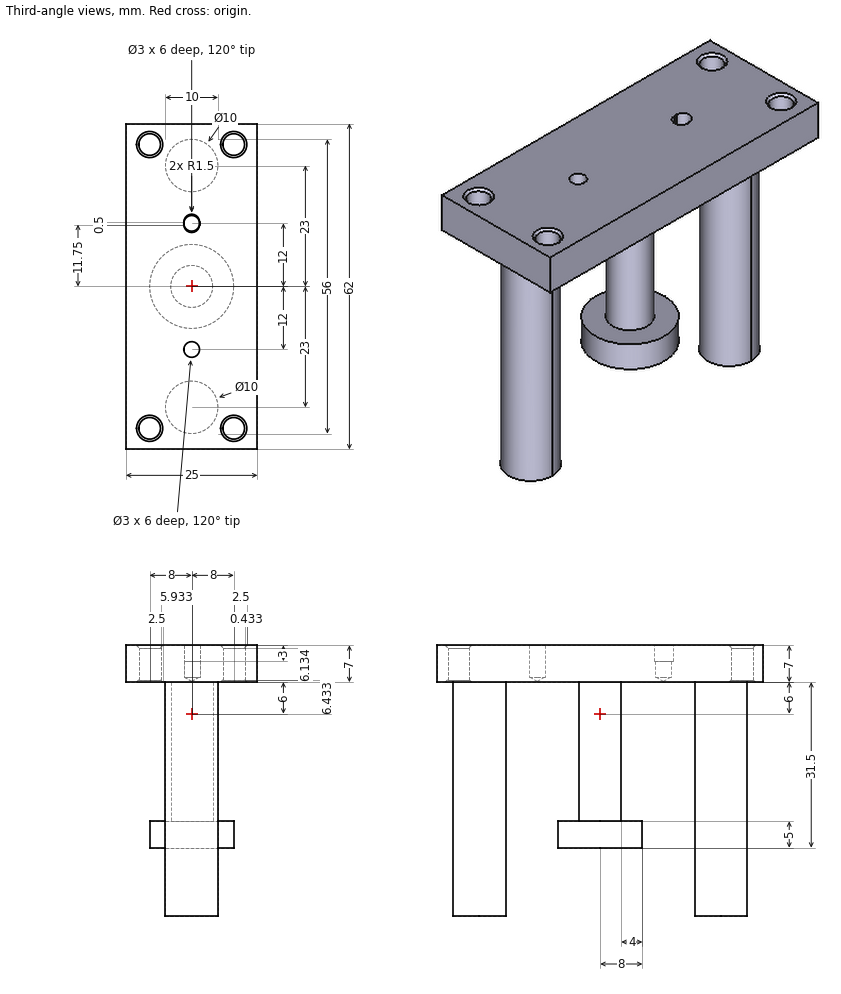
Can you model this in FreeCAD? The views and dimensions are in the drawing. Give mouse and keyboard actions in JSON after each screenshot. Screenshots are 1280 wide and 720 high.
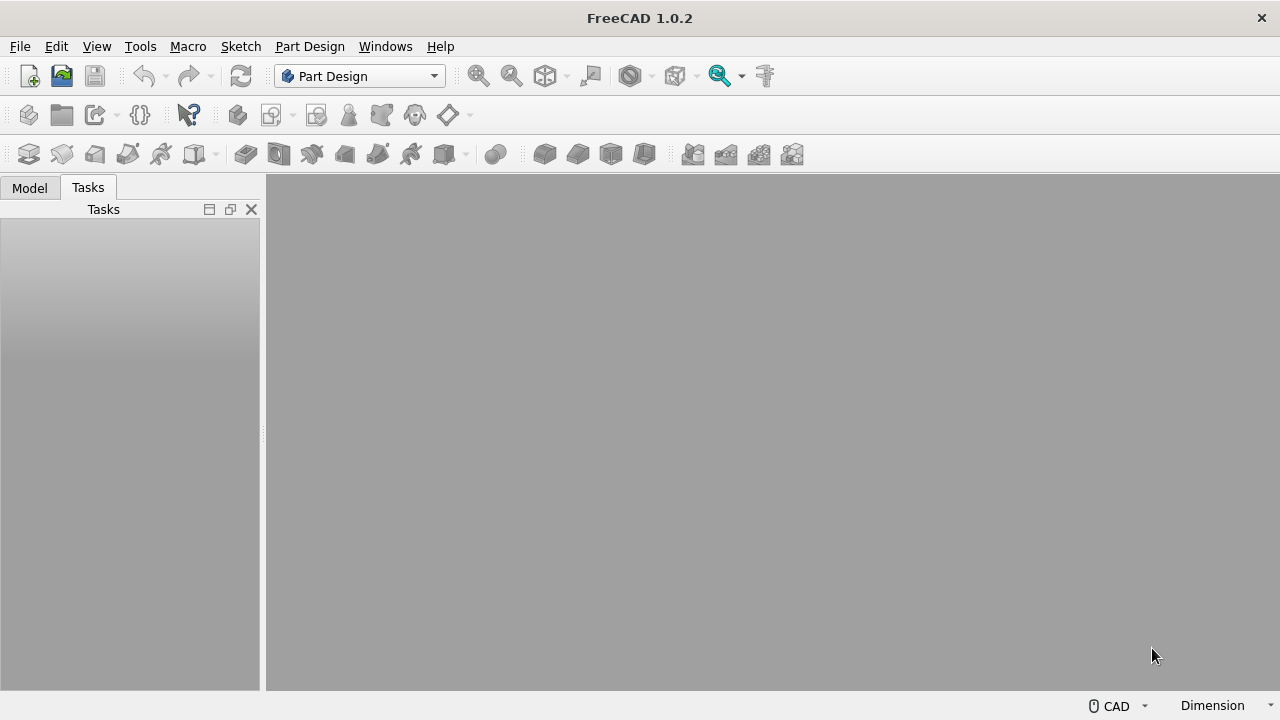
{"action": "left_click", "coordinate": [29, 76]}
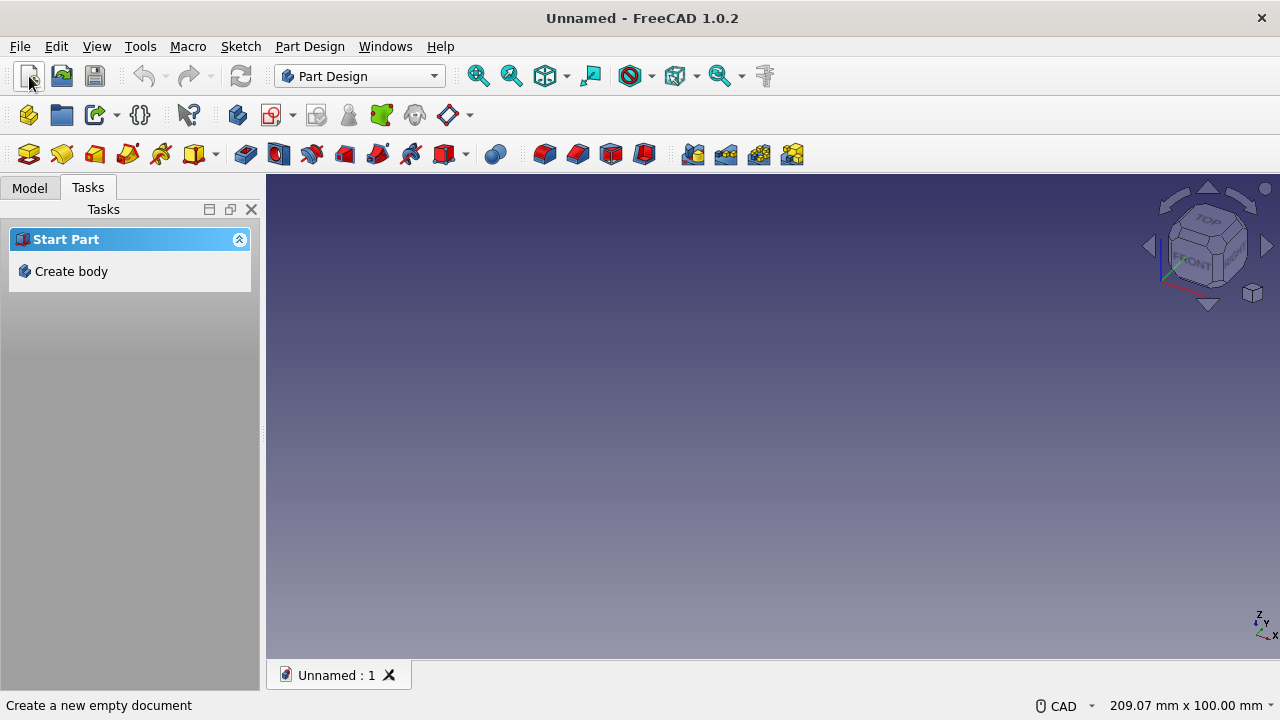
{"action": "left_click", "coordinate": [238, 116]}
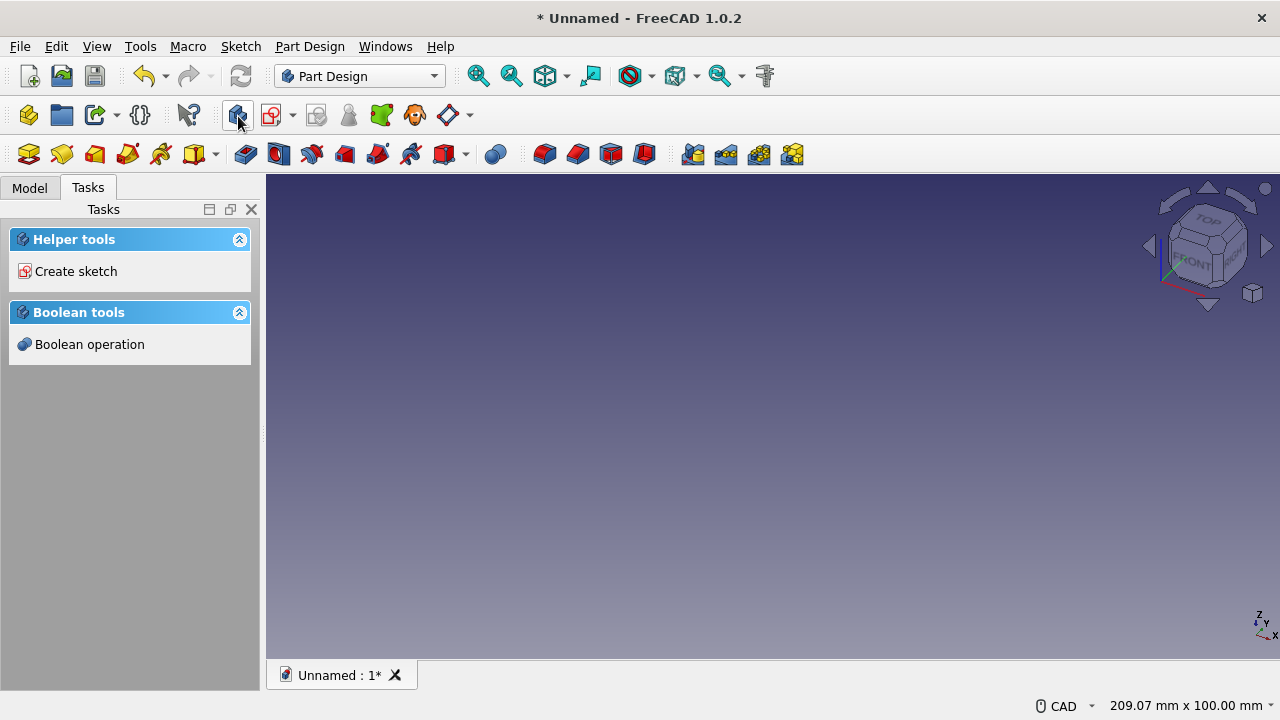
{"action": "left_click", "coordinate": [30, 188]}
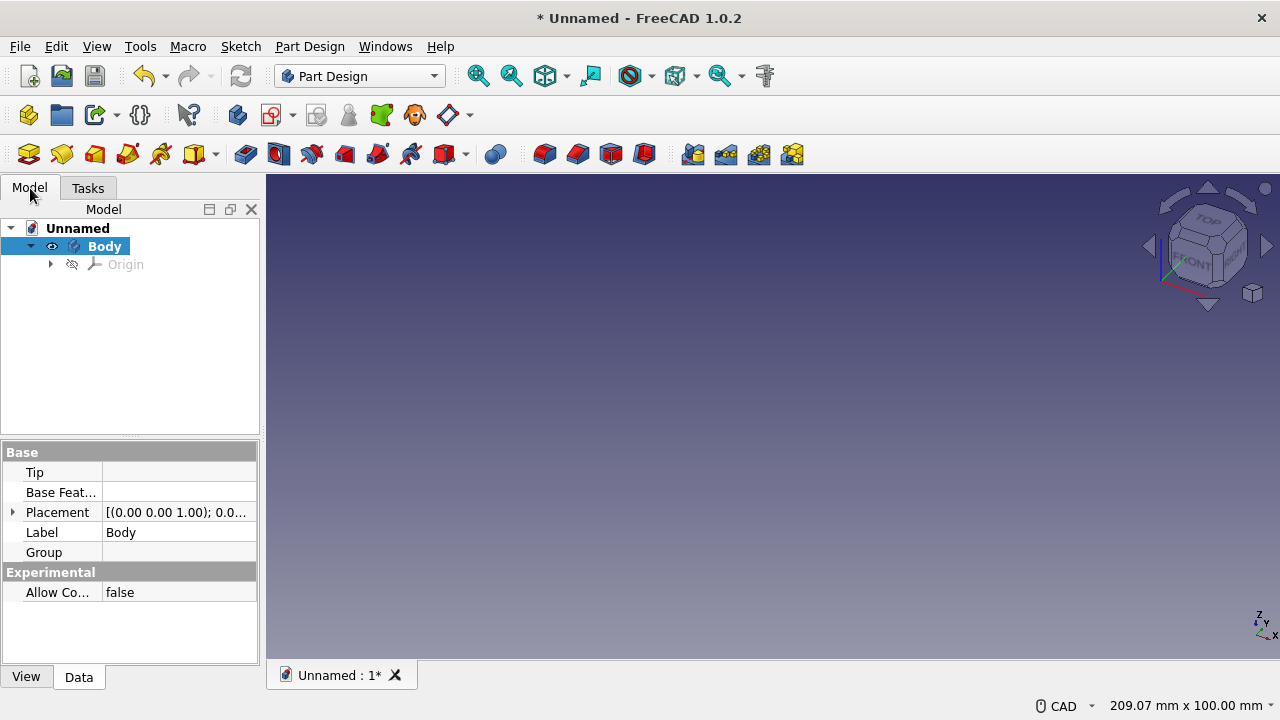
{"action": "left_click", "coordinate": [51, 264]}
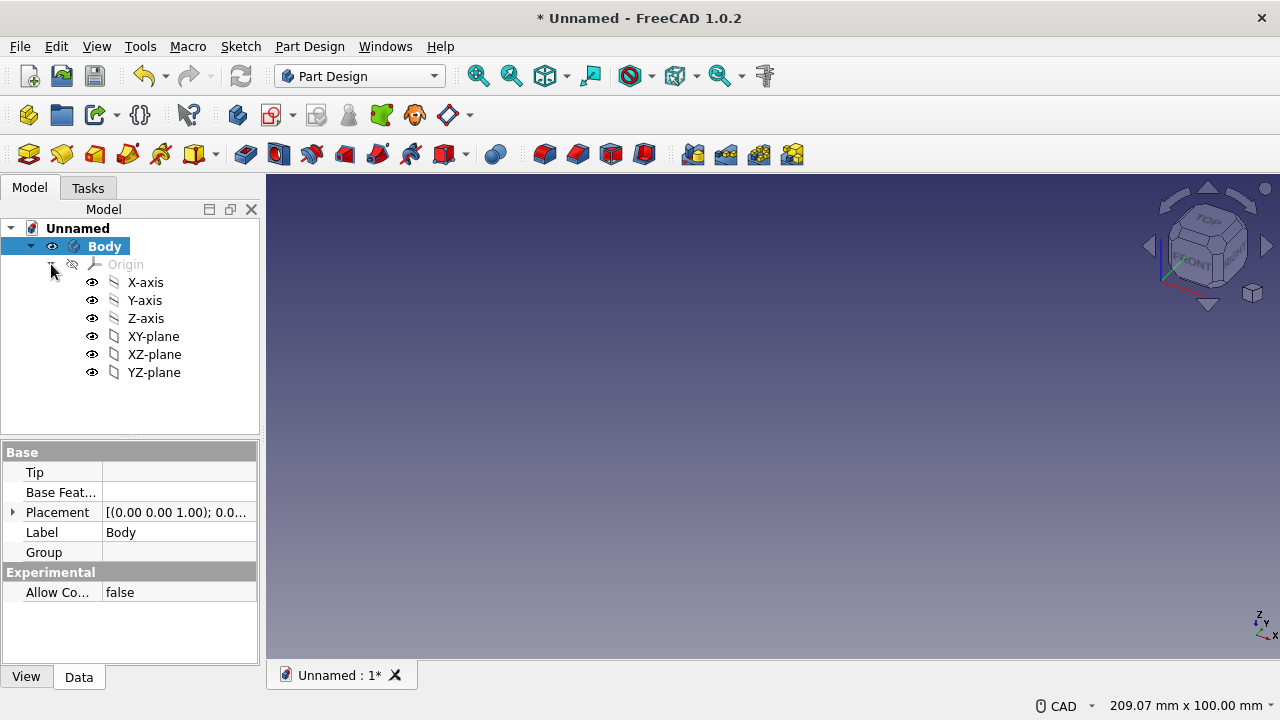
{"action": "left_click", "coordinate": [137, 336]}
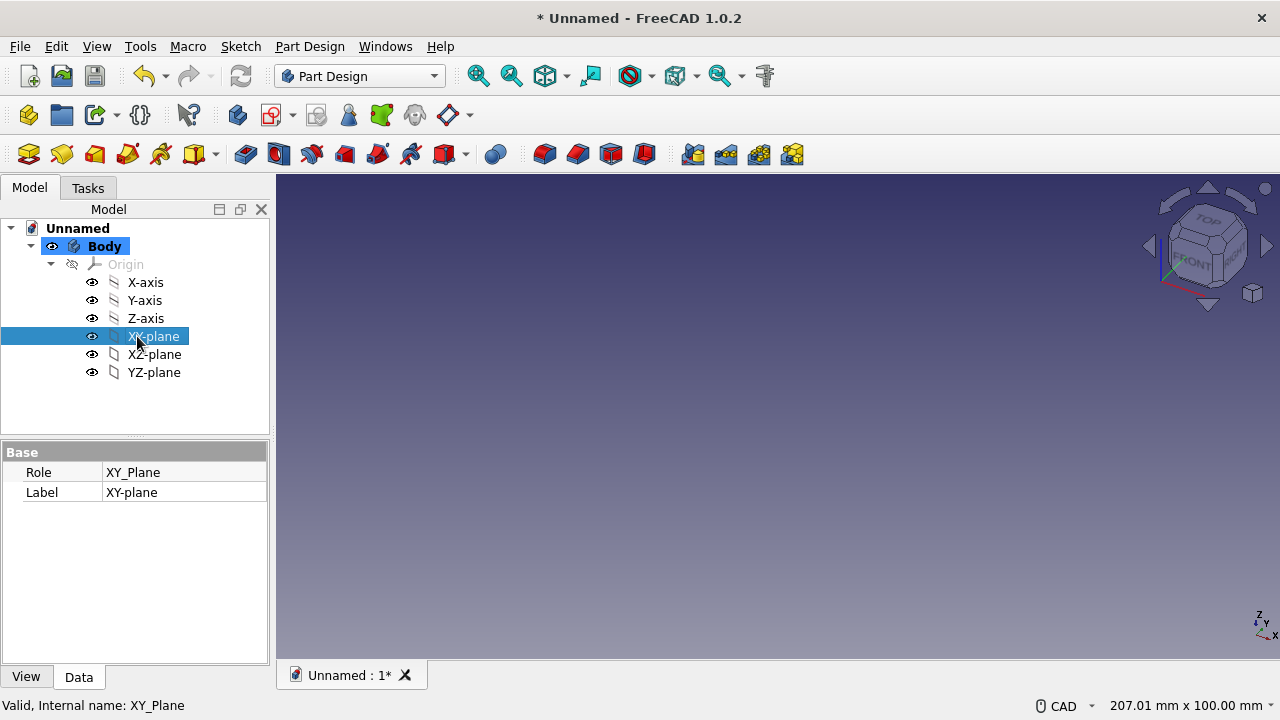
{"action": "left_click", "coordinate": [448, 116]}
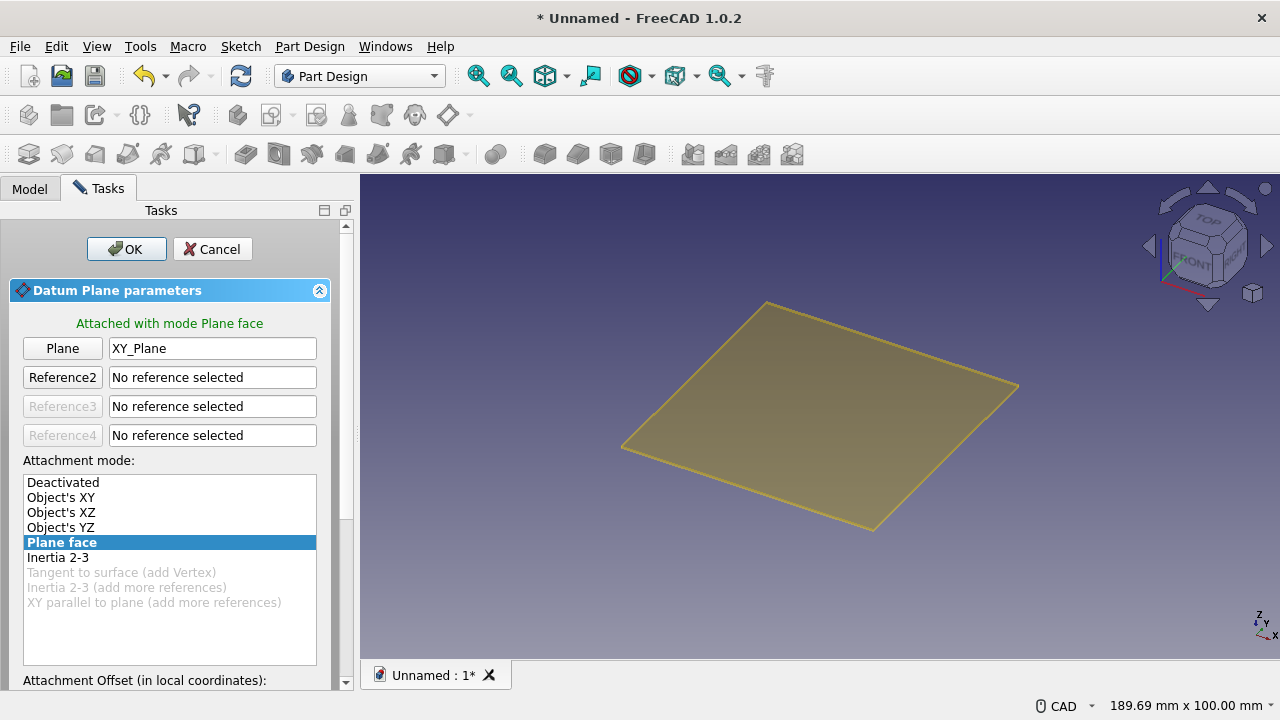
{"action": "scroll", "coordinate": [346, 455], "scroll_direction": "down", "scroll_amount": 3}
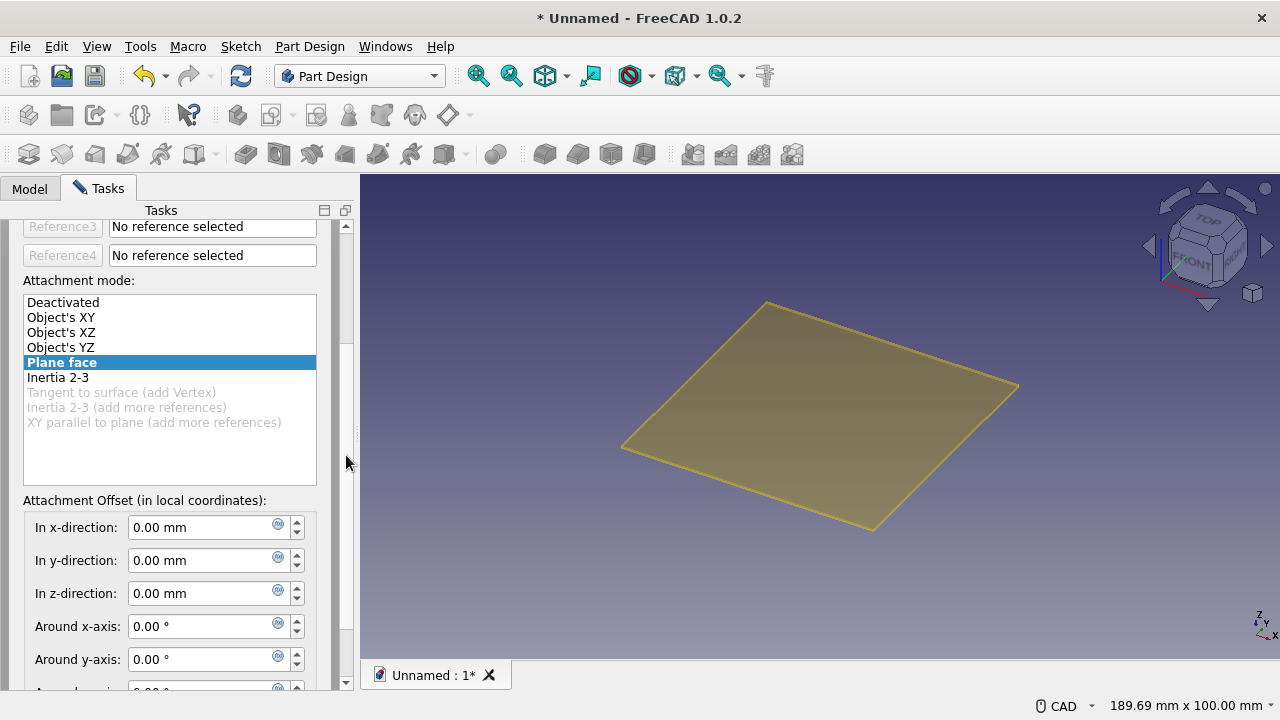
{"action": "triple_click", "coordinate": [210, 594]}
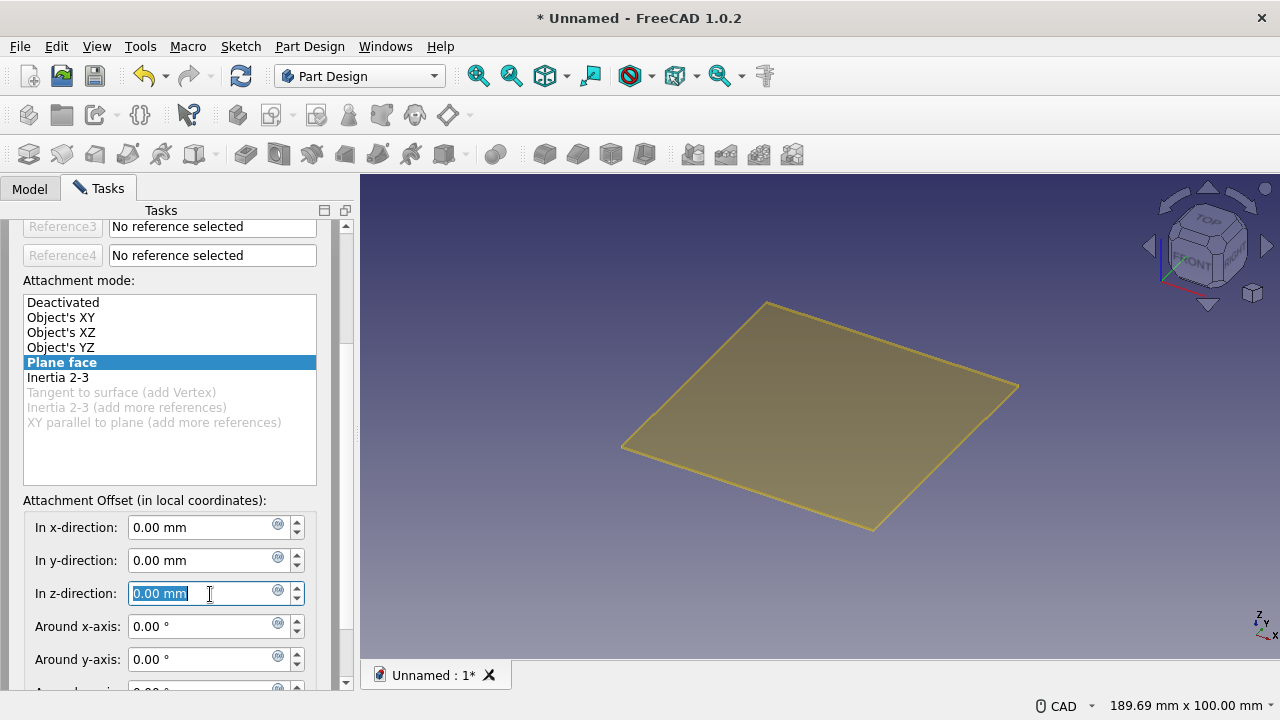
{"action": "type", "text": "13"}
{"action": "key", "text": "Tab"}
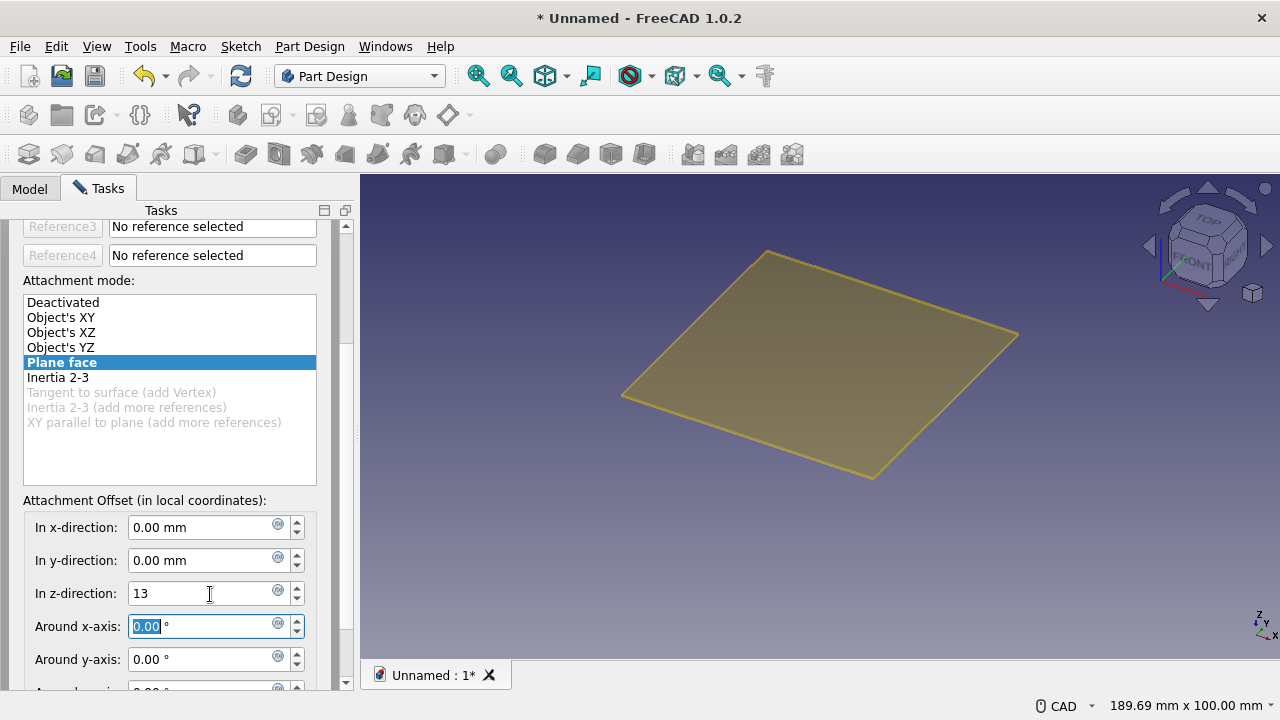
{"action": "scroll", "coordinate": [346, 455], "scroll_direction": "up", "scroll_amount": 4}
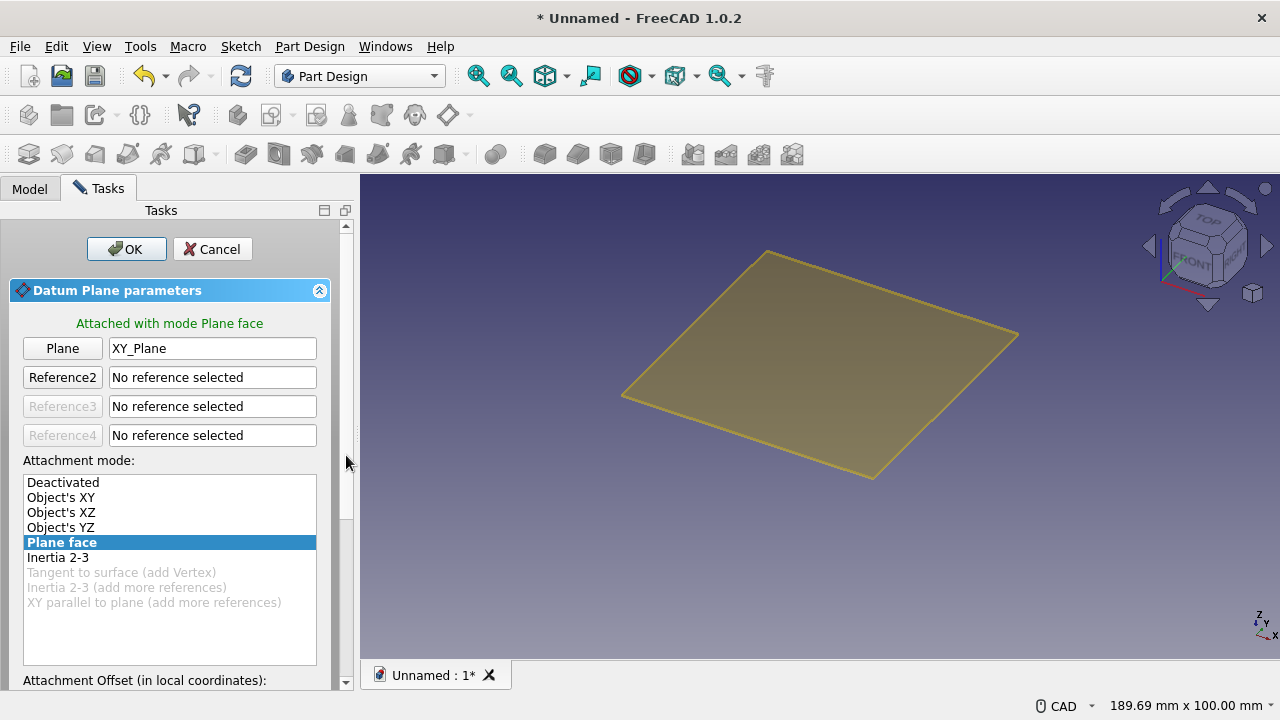
{"action": "left_click", "coordinate": [127, 249]}